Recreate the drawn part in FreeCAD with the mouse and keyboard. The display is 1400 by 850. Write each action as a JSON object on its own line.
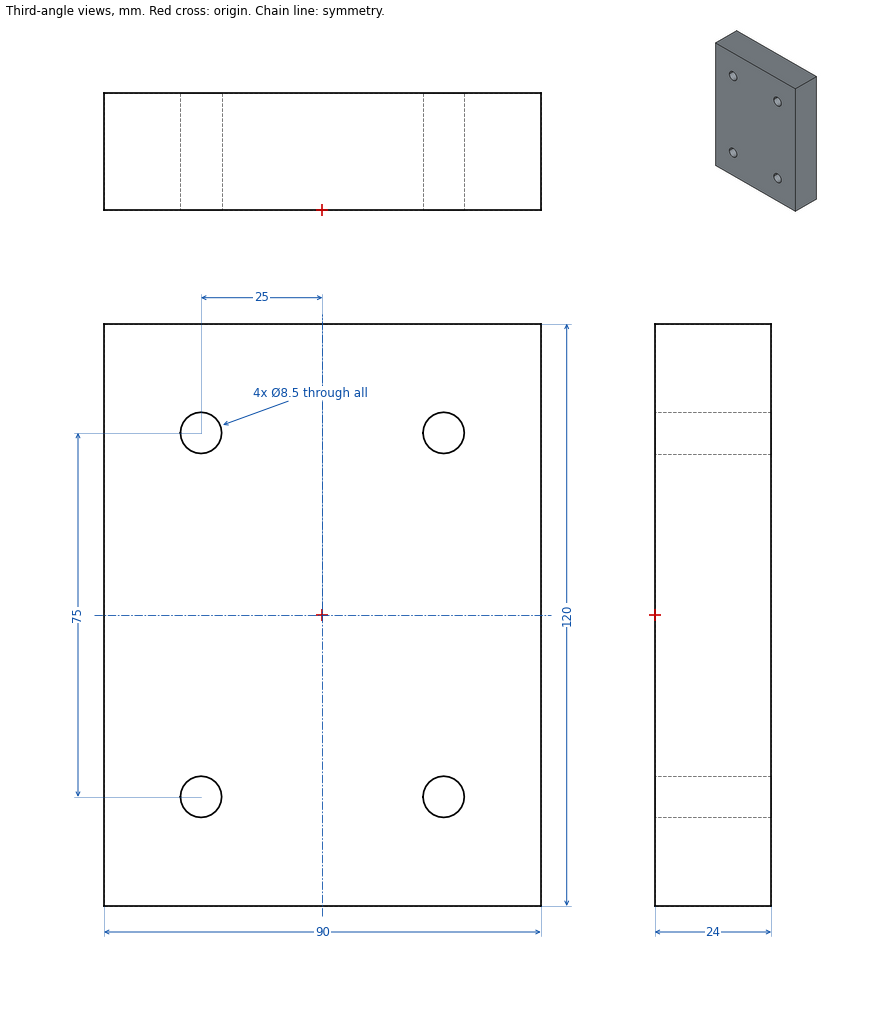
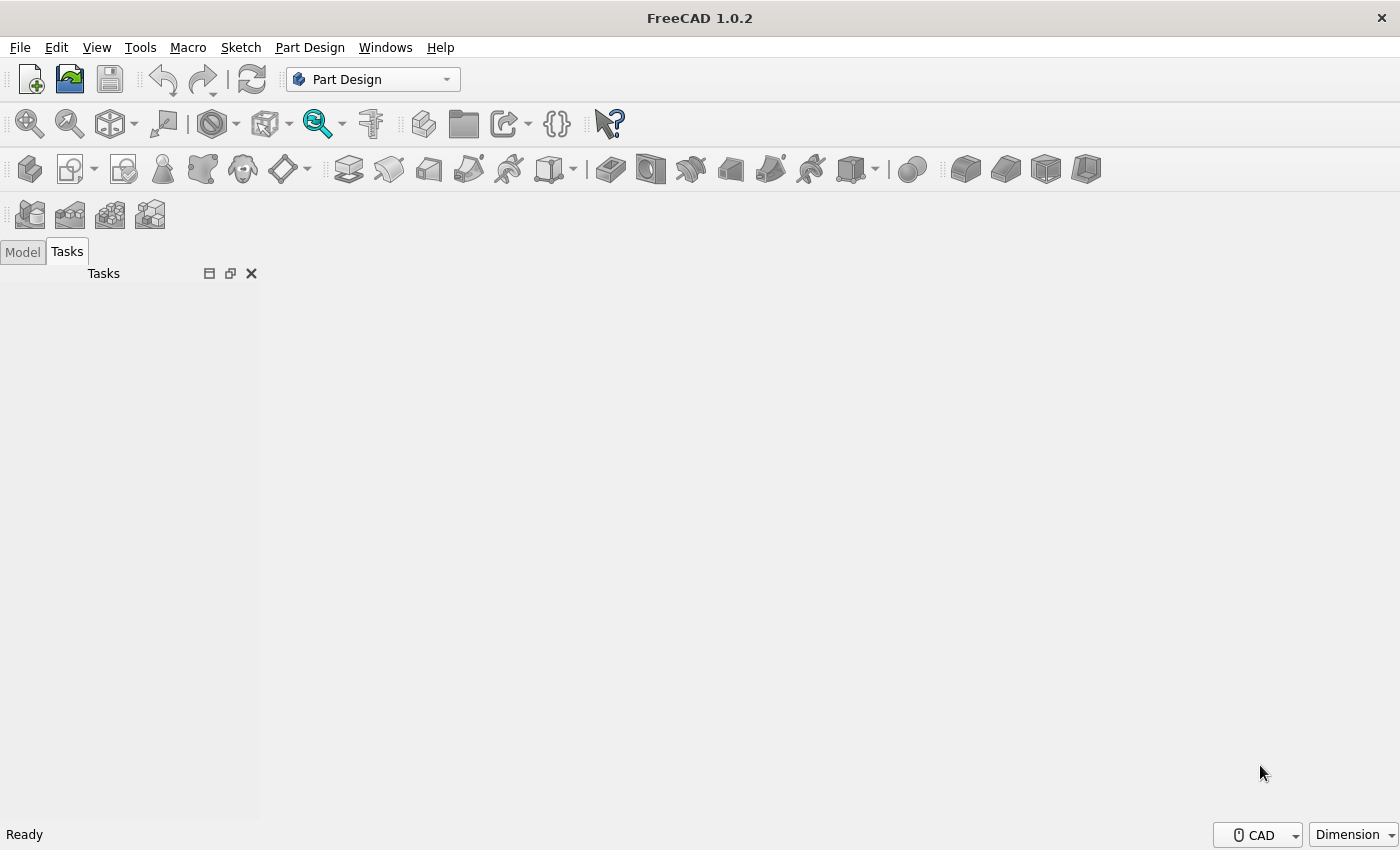
{"action": "left_click", "coordinate": [30, 80]}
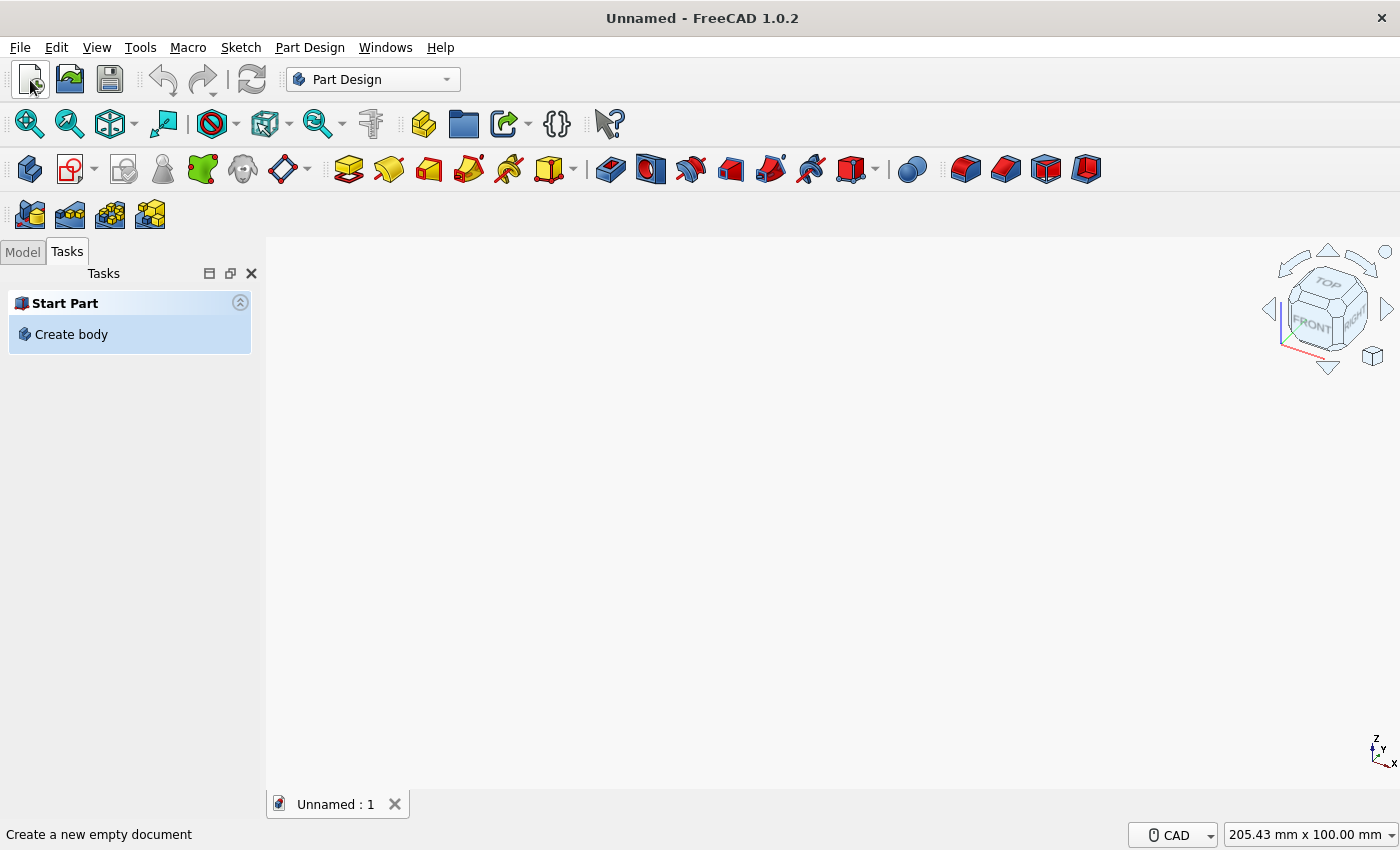
{"action": "left_click", "coordinate": [70, 170]}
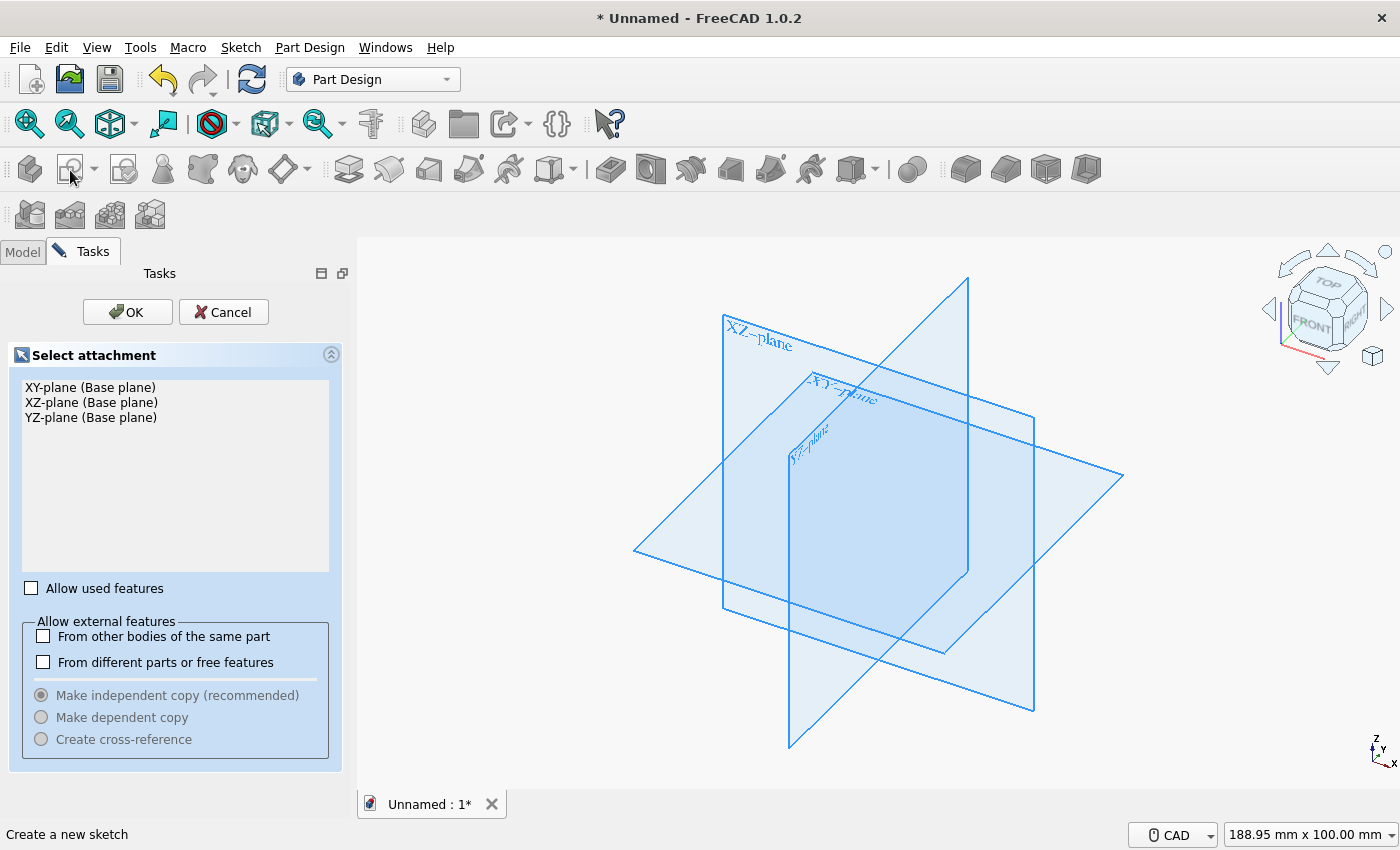
{"action": "left_click", "coordinate": [82, 402]}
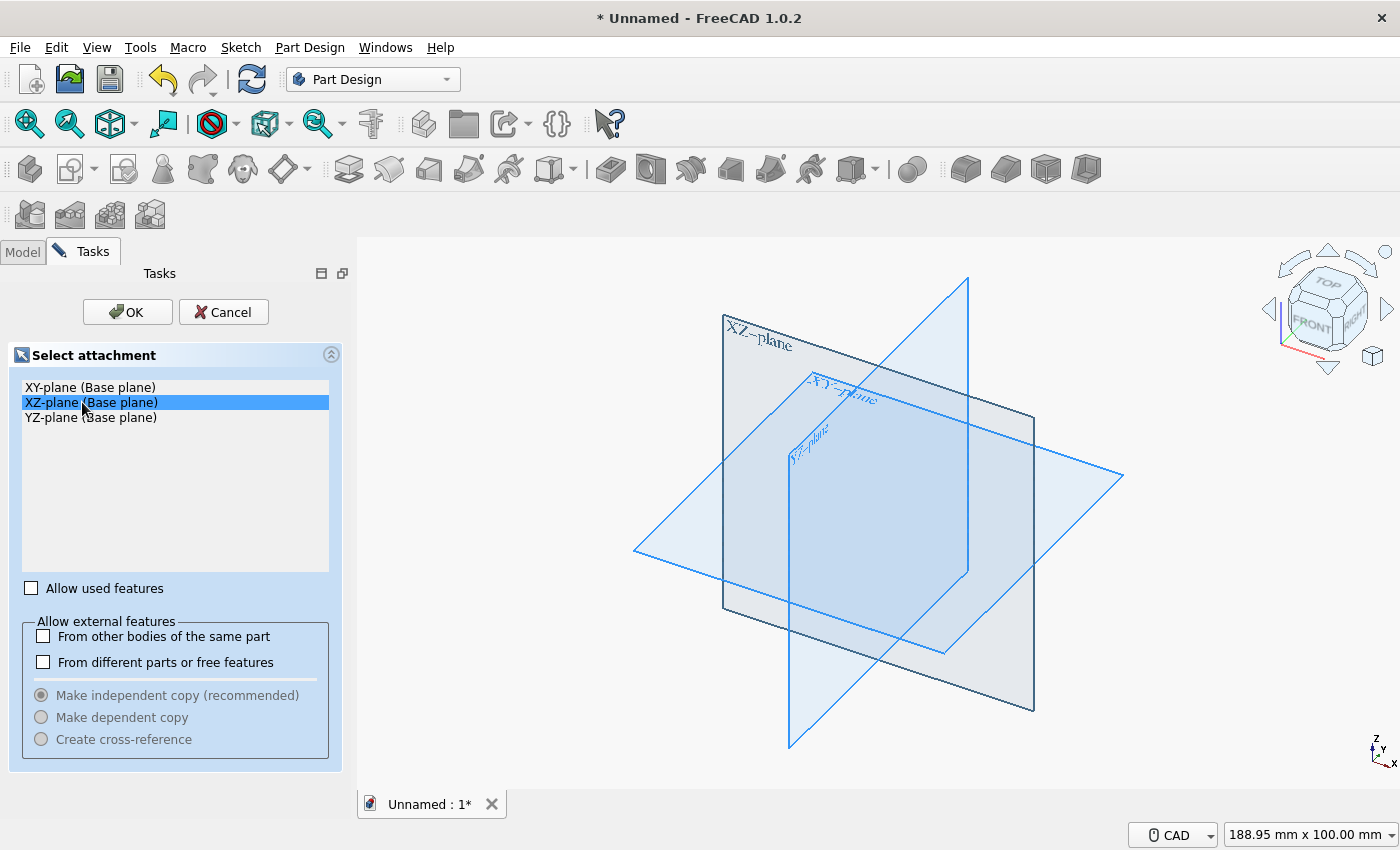
{"action": "left_click", "coordinate": [128, 312]}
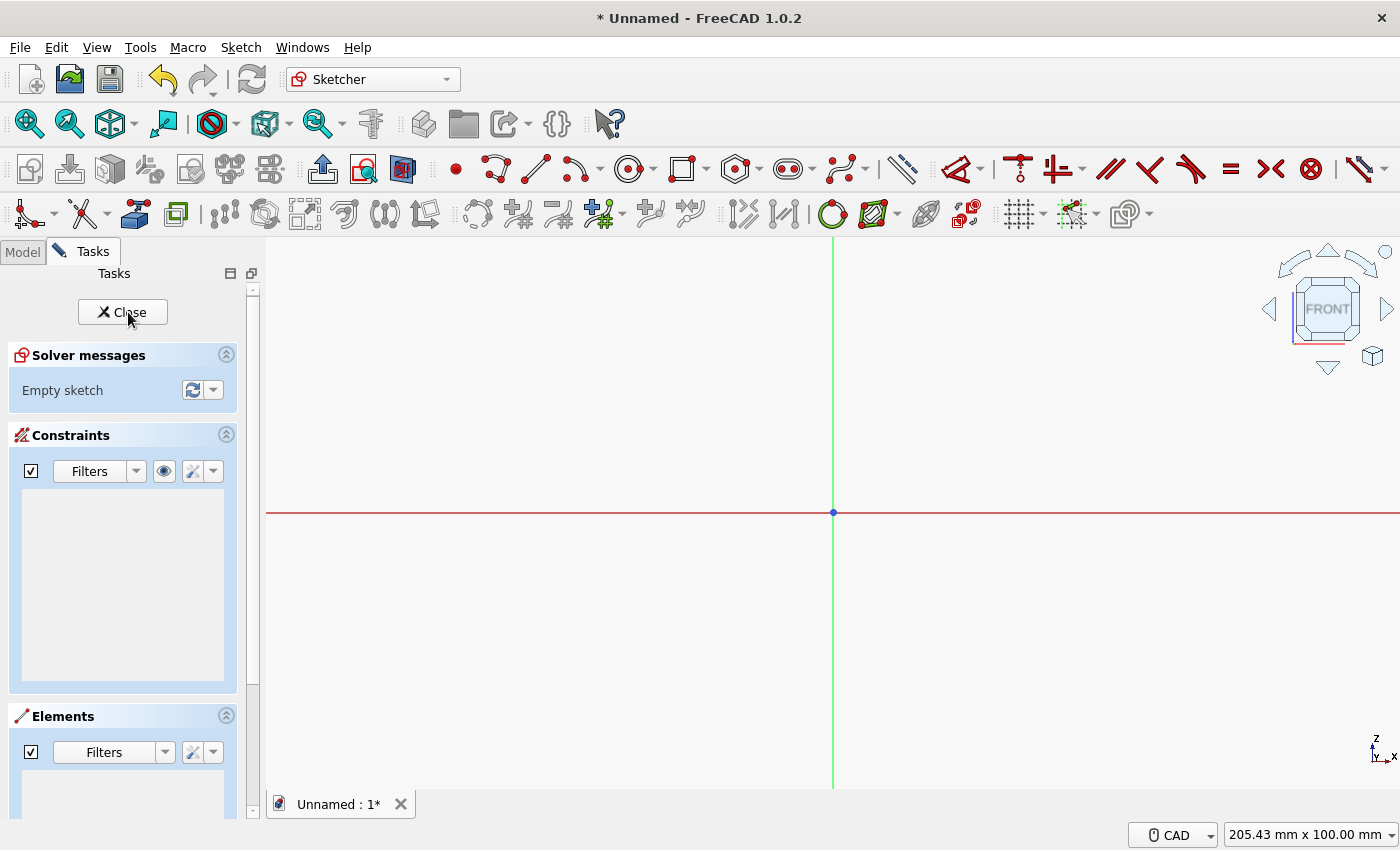
{"action": "scroll", "coordinate": [681, 513], "scroll_direction": "down", "scroll_amount": 3}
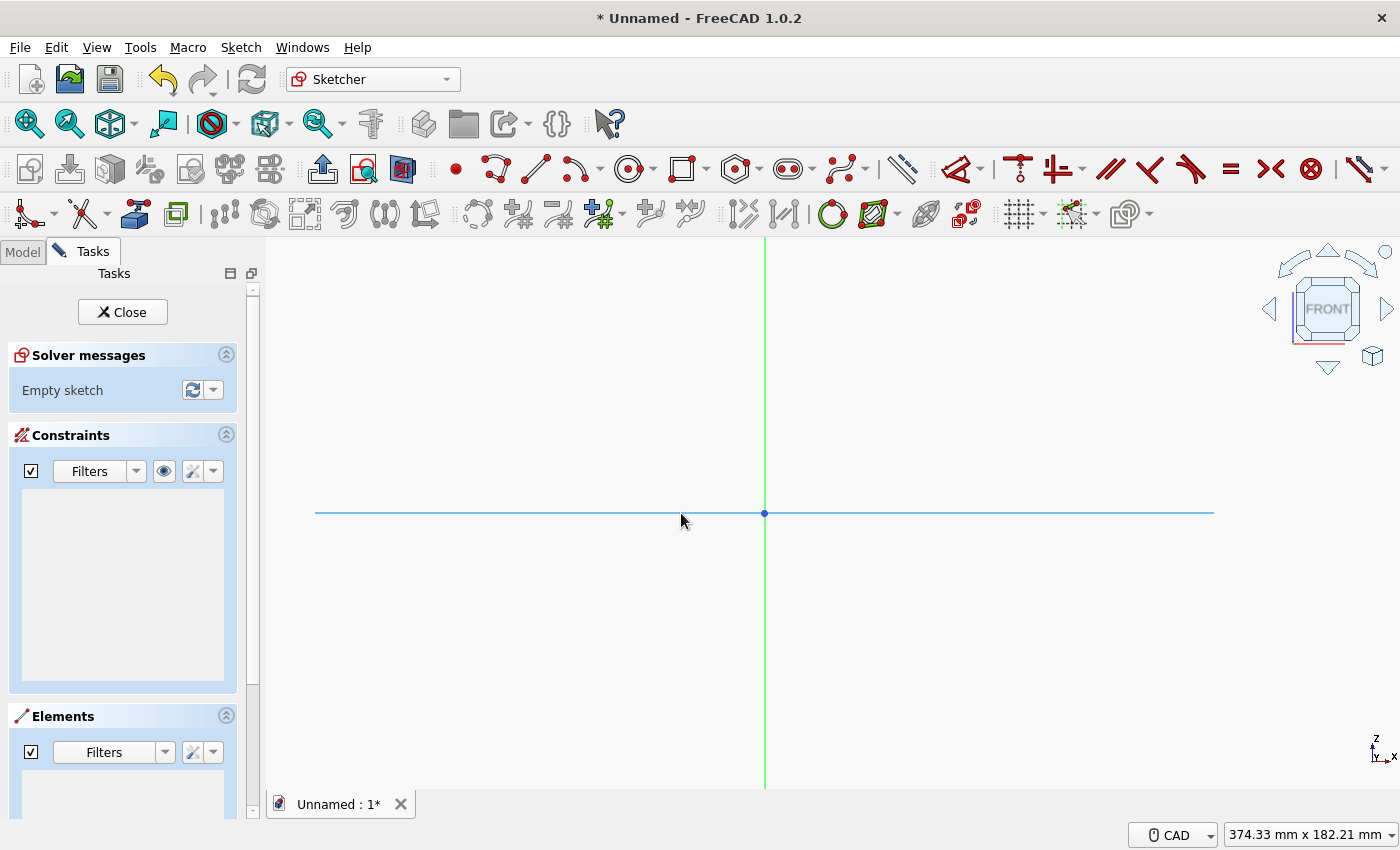
{"action": "key", "text": "g v"}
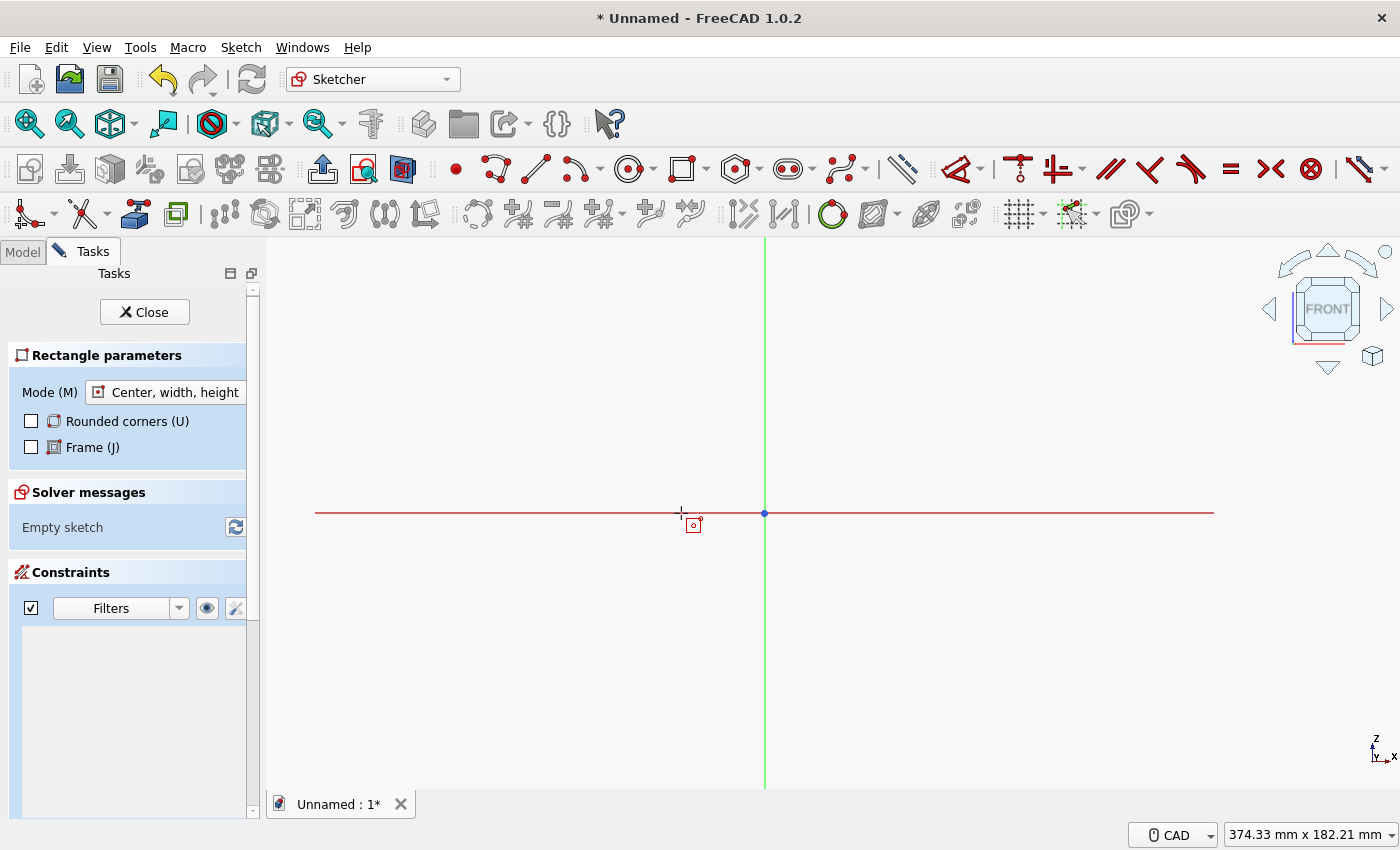
{"action": "left_click", "coordinate": [765, 513]}
{"action": "left_click", "coordinate": [901, 331]}
{"action": "key", "text": "Escape"}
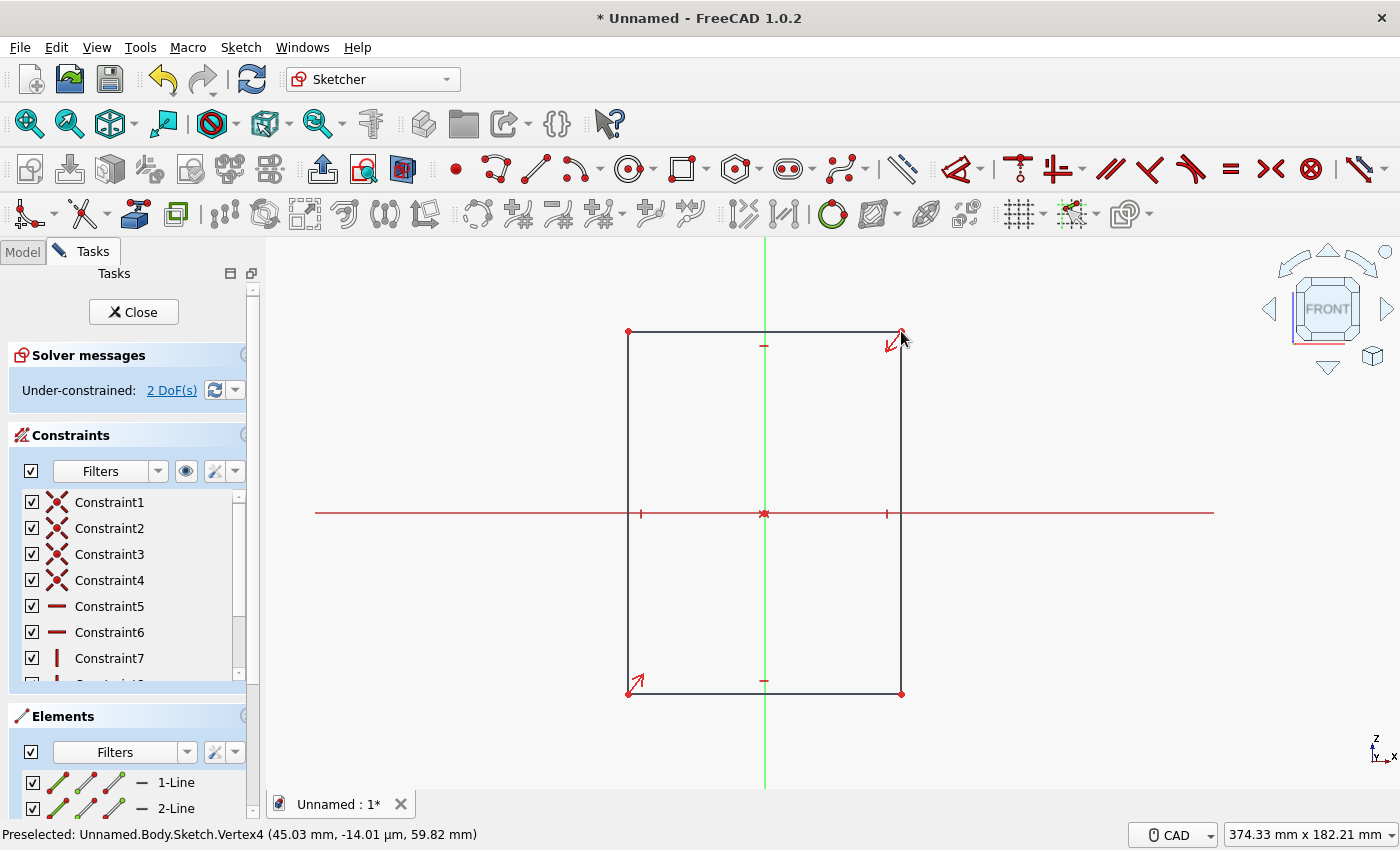
{"action": "left_click", "coordinate": [710, 694]}